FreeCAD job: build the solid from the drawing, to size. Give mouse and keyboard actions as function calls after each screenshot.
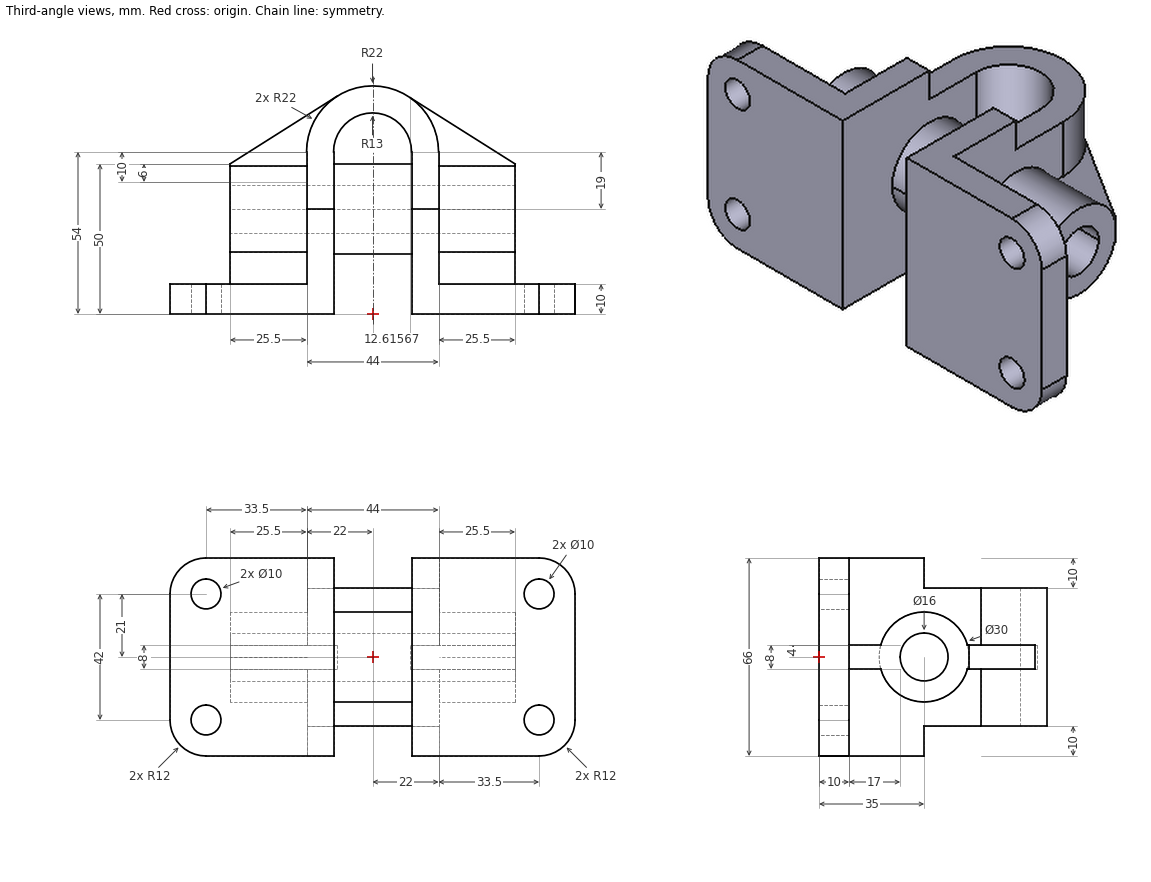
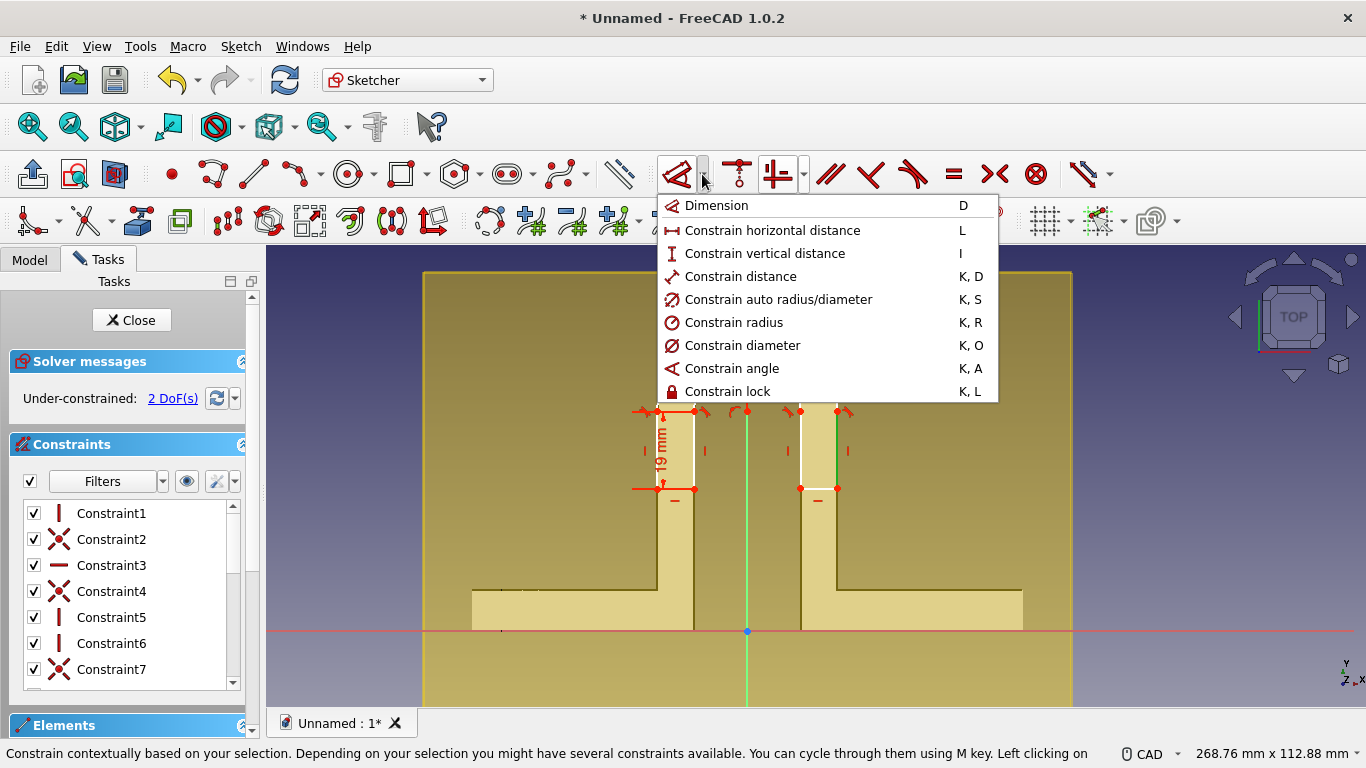
click(828, 254)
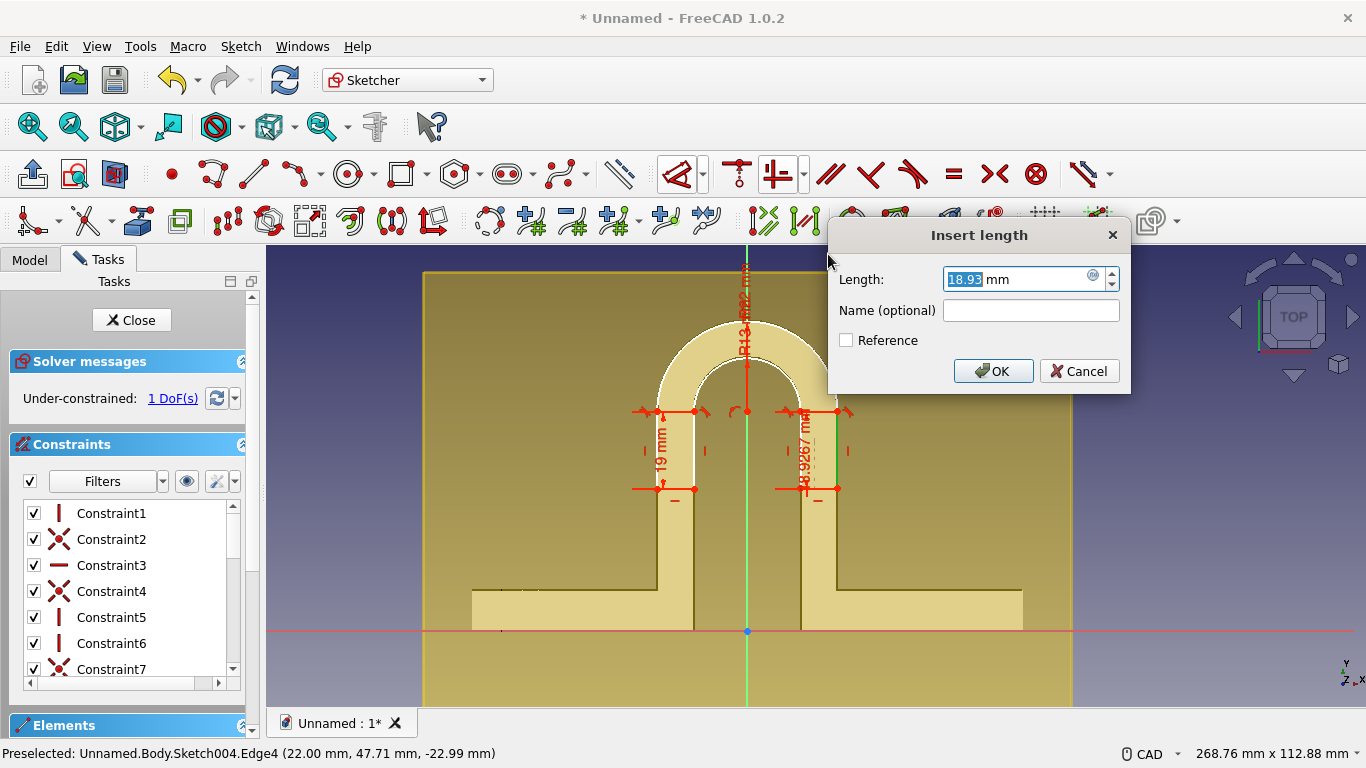
text(19)
key(Return)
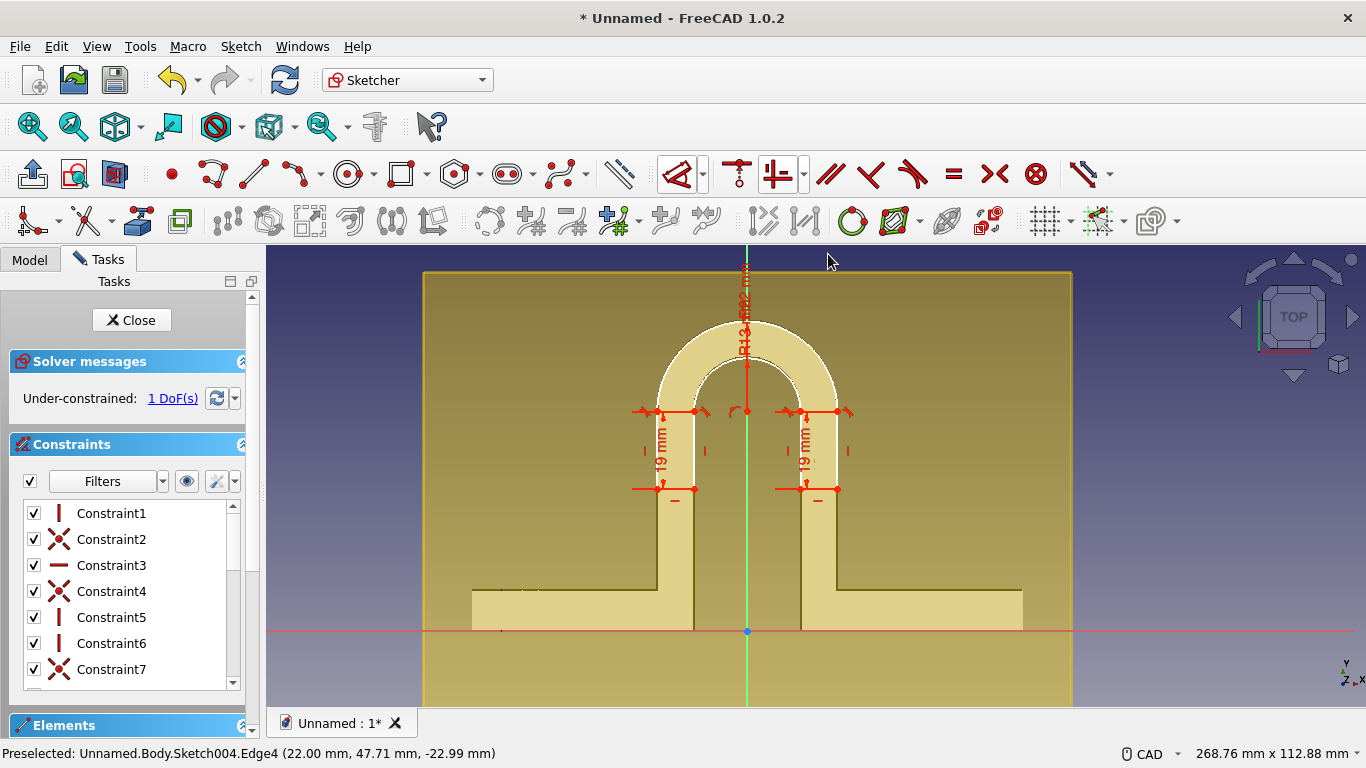
click(694, 412)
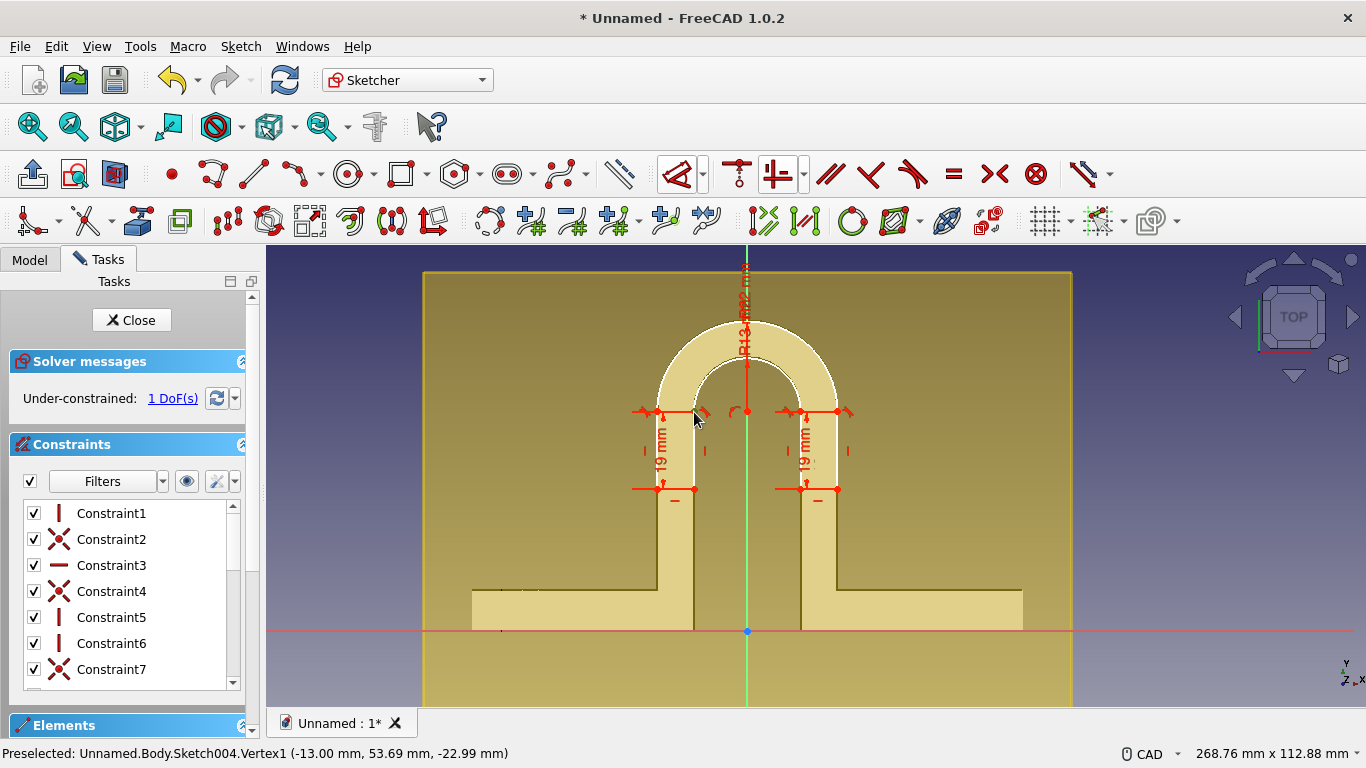
key(i)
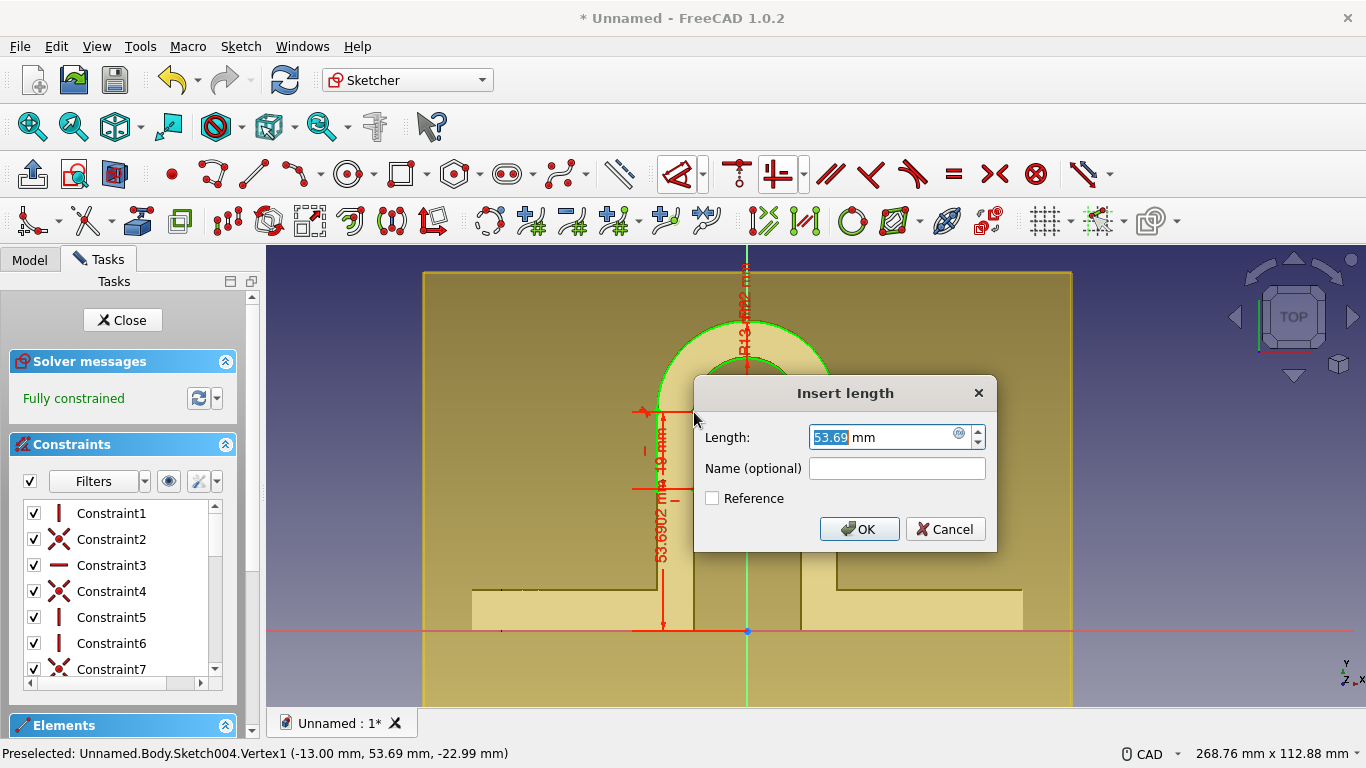
text(54)
key(Return)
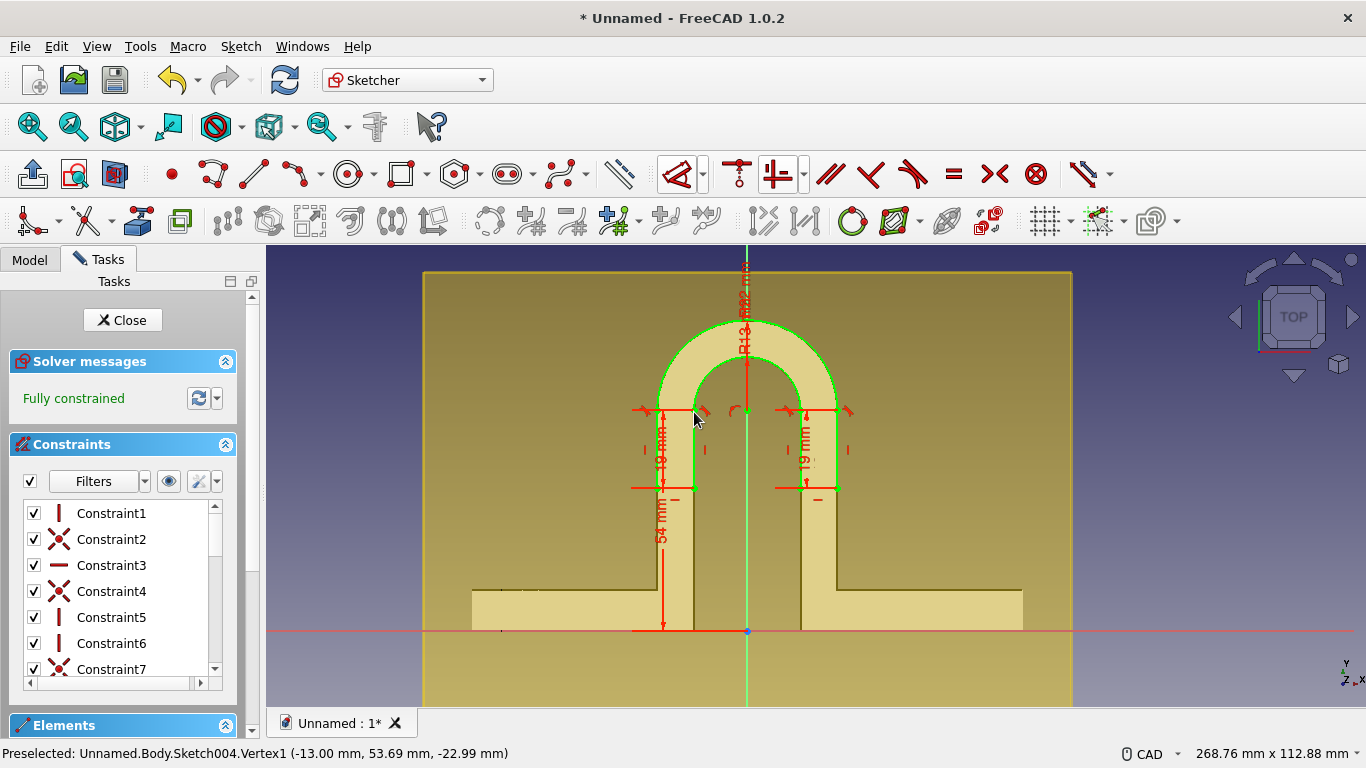
click(123, 320)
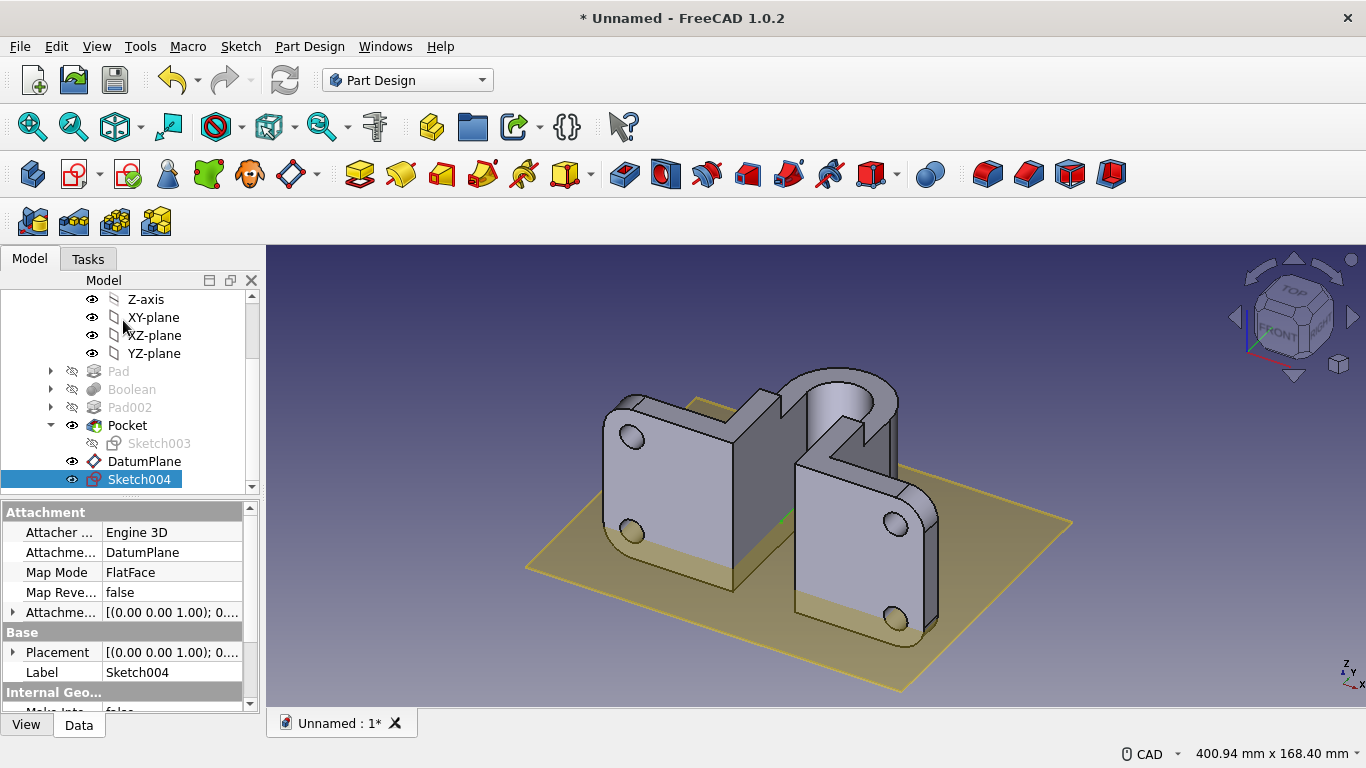
click(625, 174)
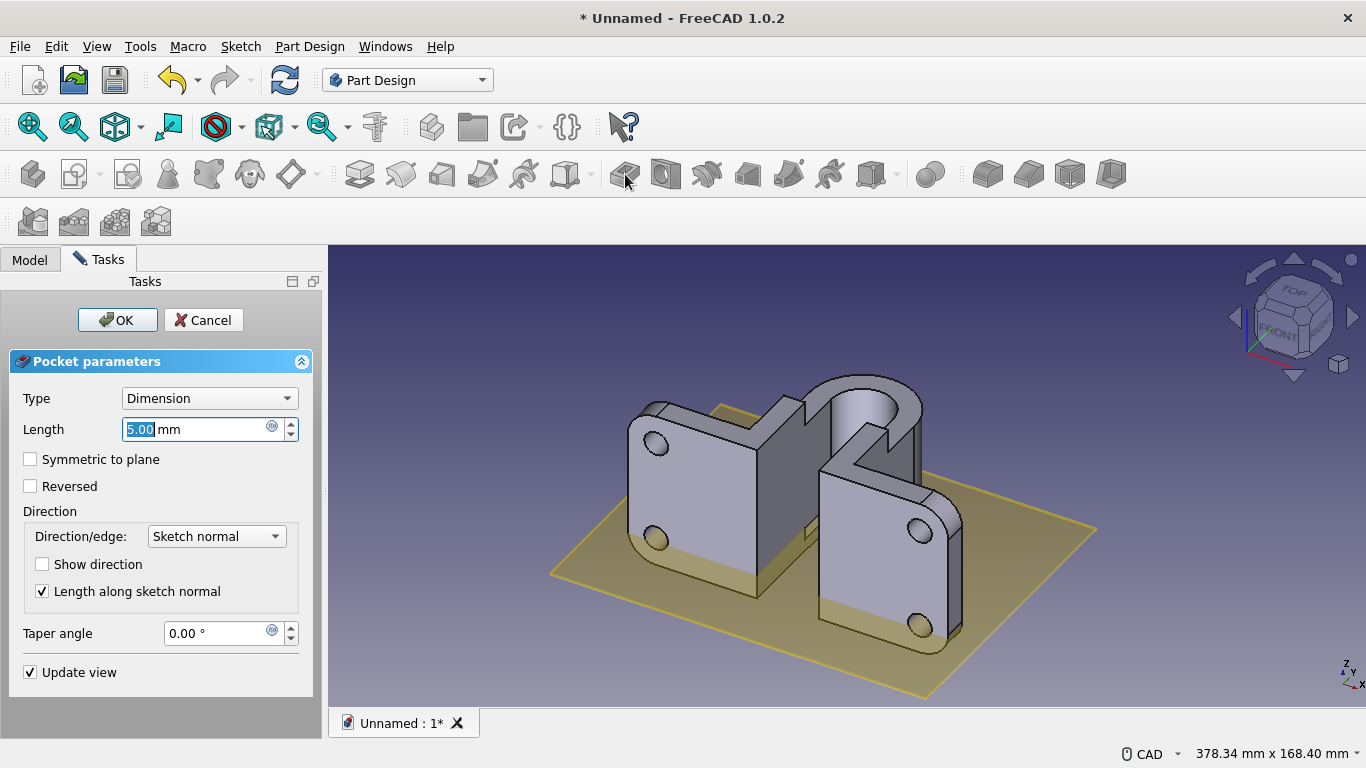
text(10)
key(Tab)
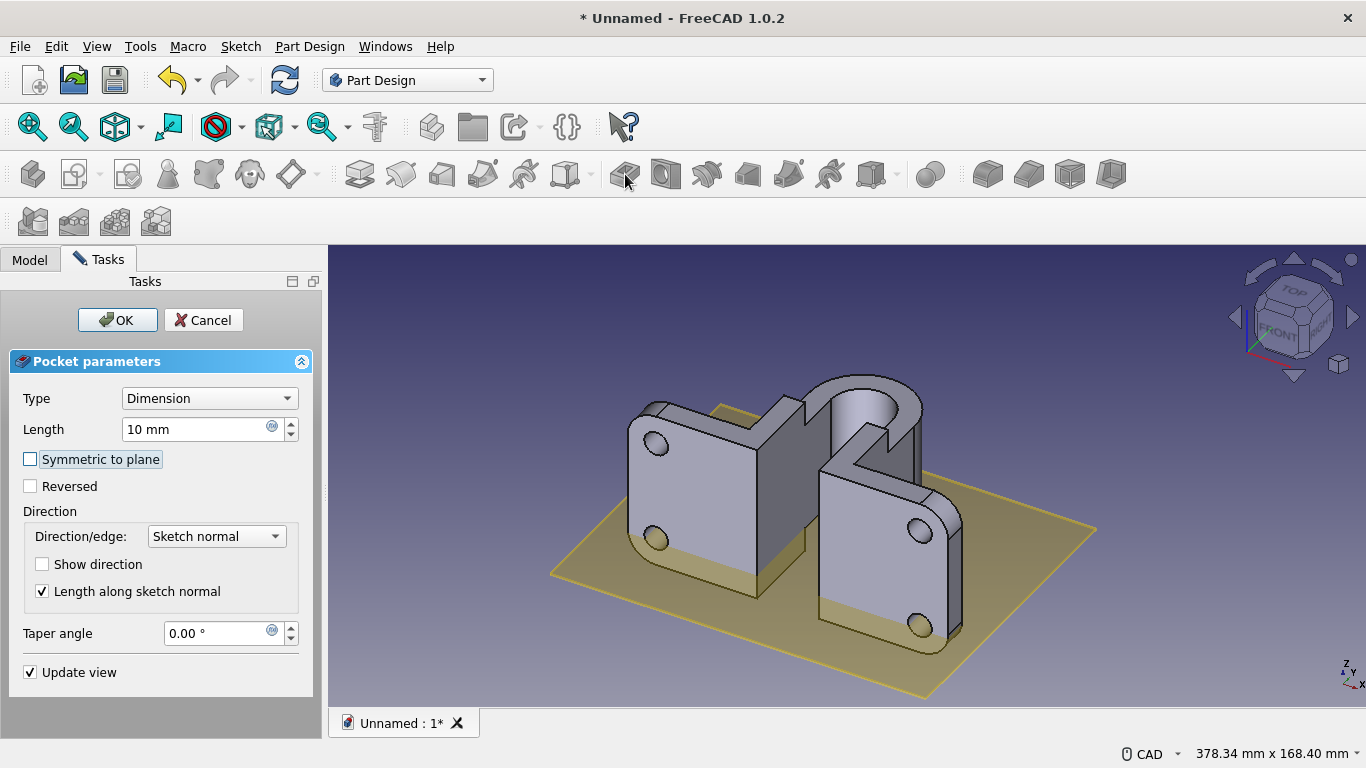
click(118, 320)